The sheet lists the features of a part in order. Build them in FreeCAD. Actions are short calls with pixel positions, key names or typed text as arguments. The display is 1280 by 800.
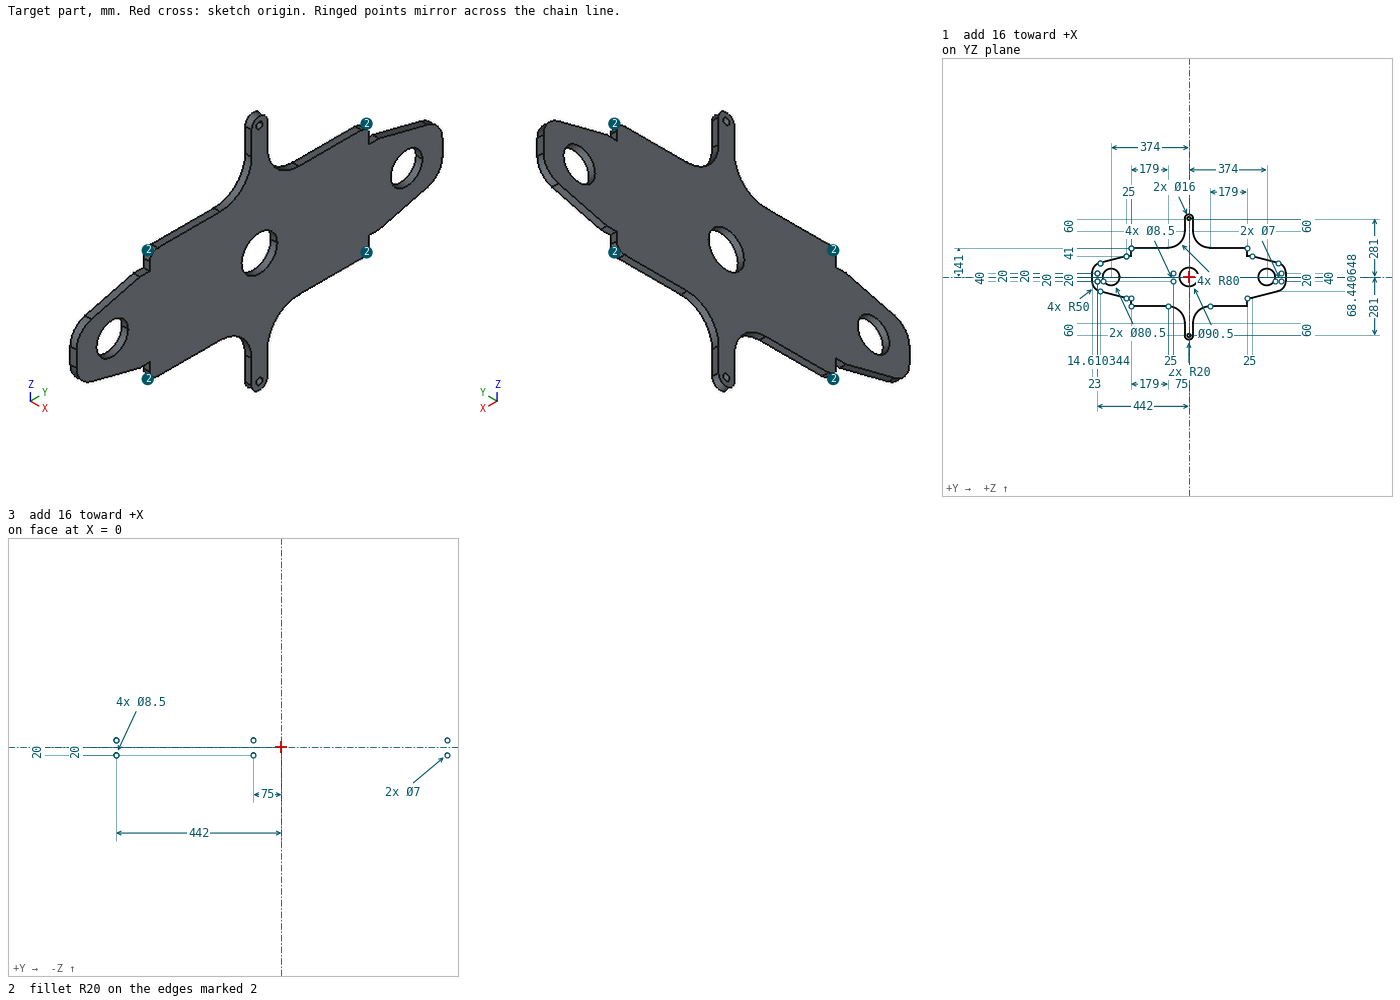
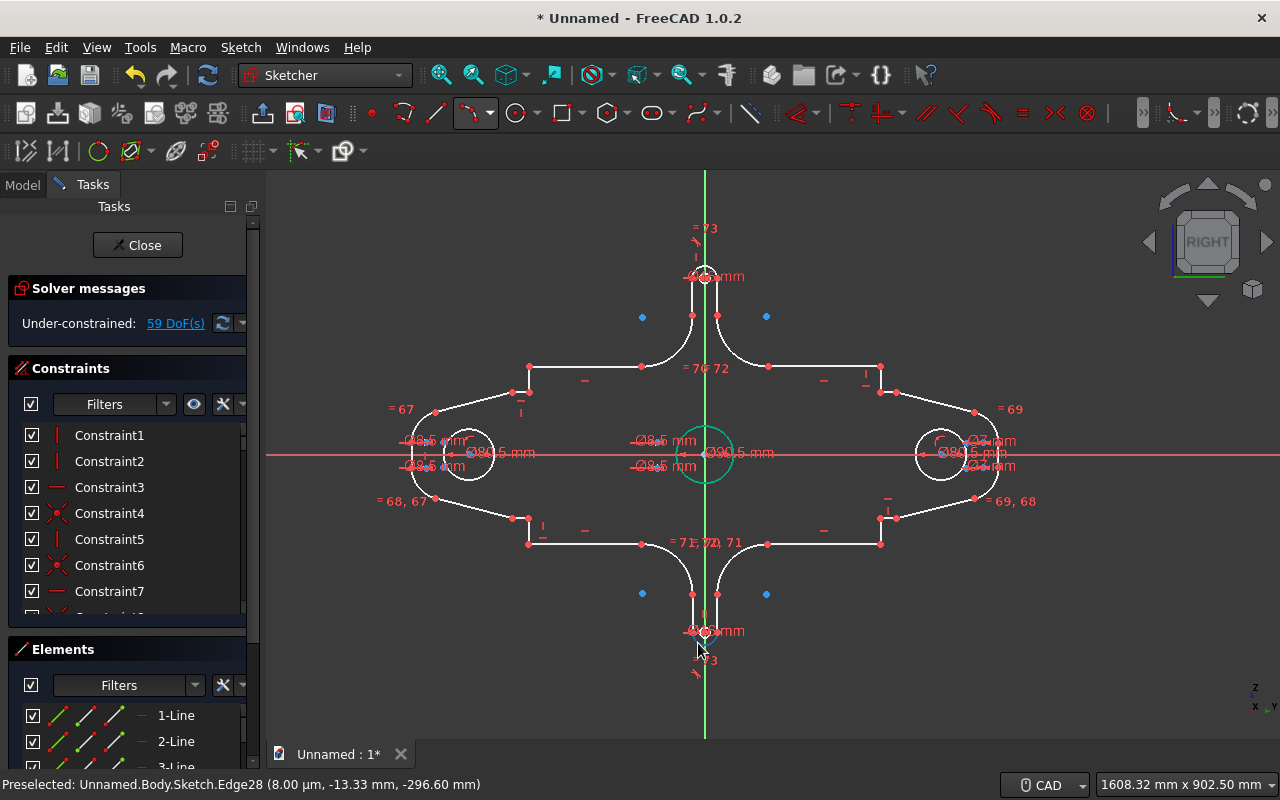
click(705, 278)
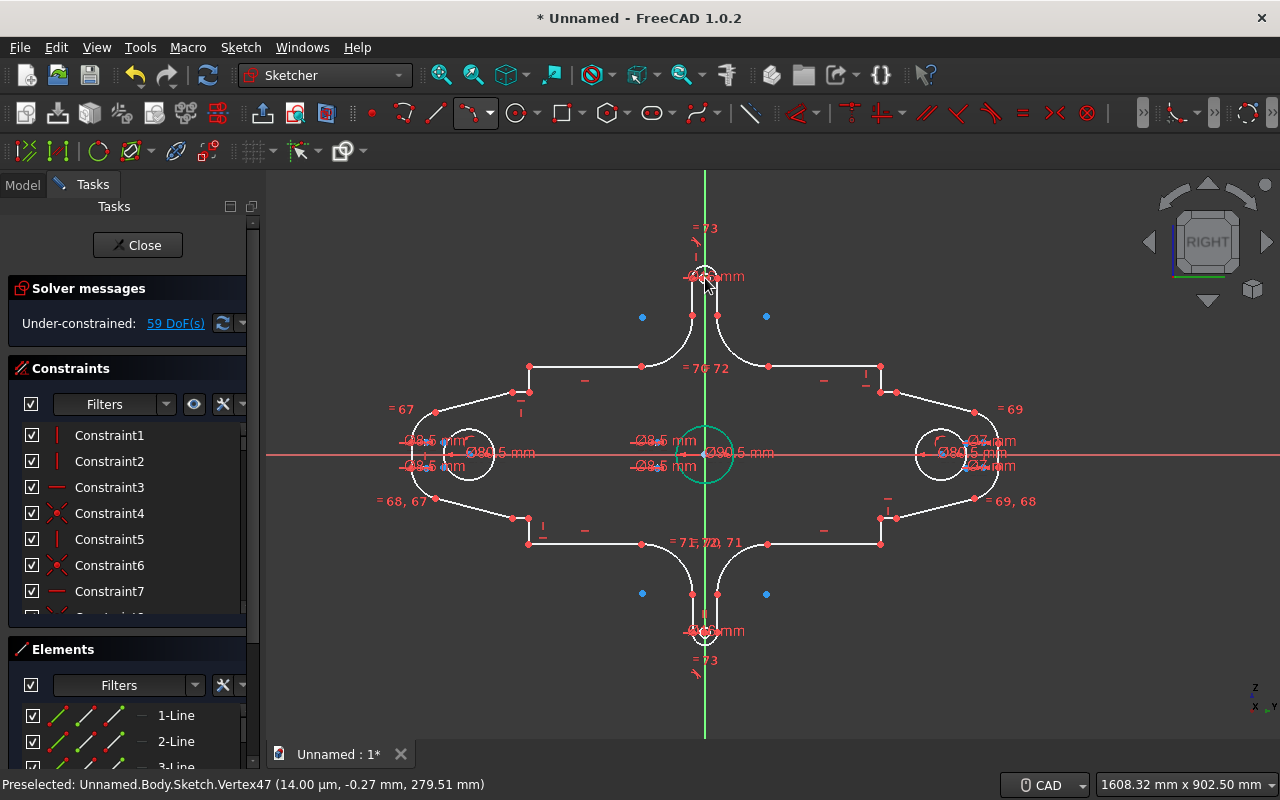
click(705, 528)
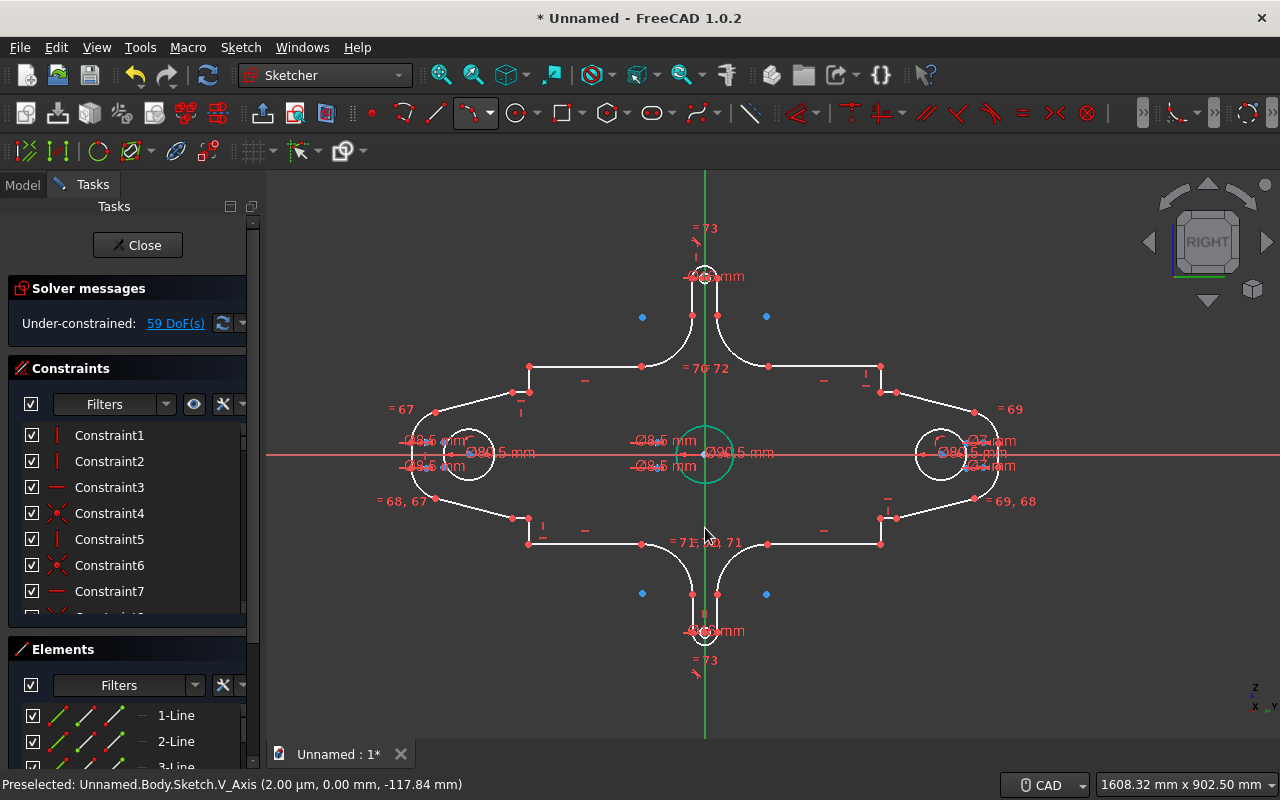
click(850, 114)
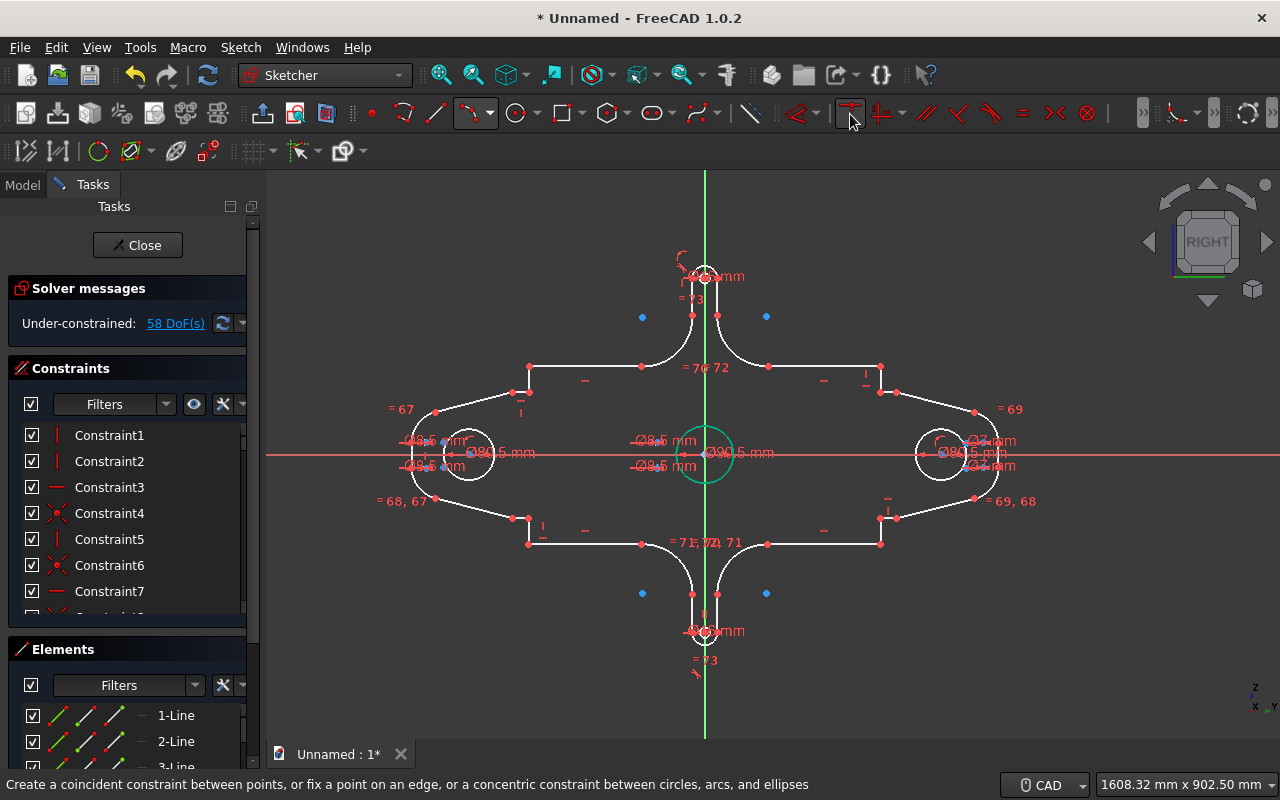
click(705, 633)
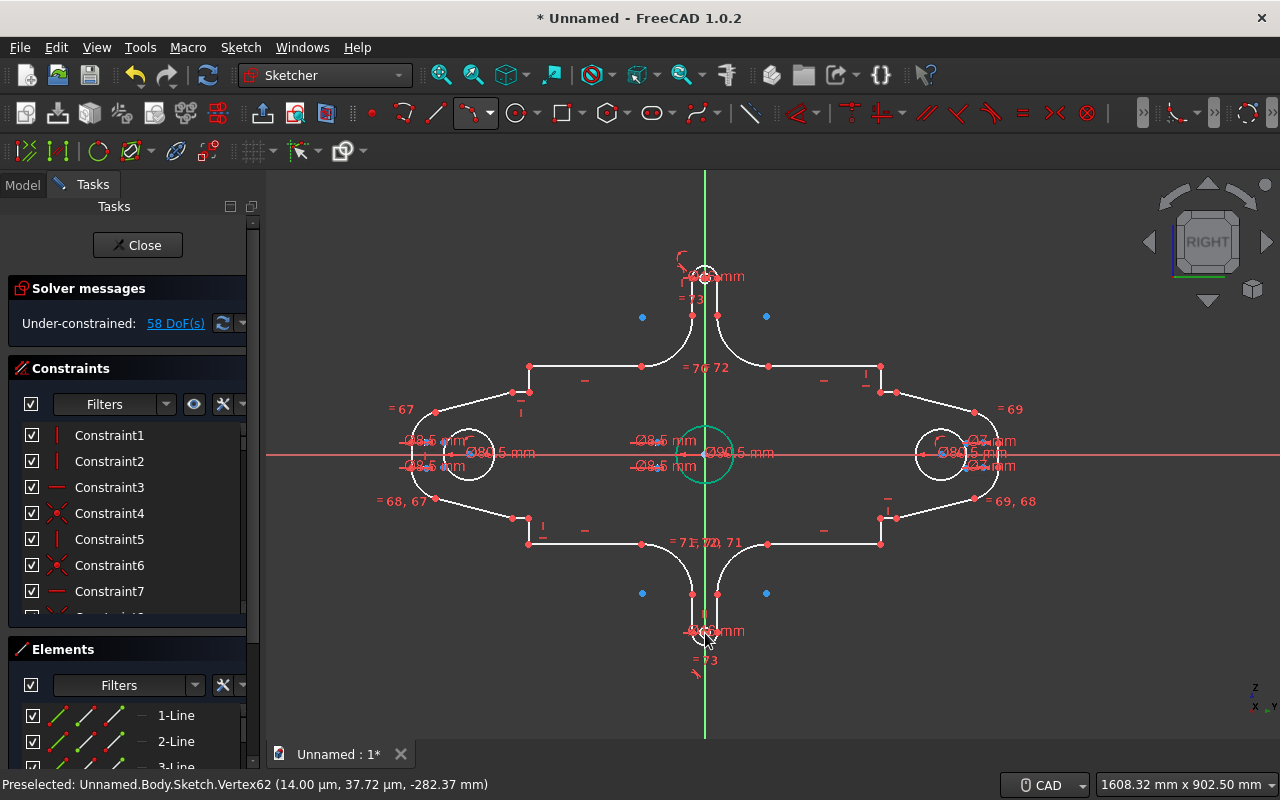
click(705, 528)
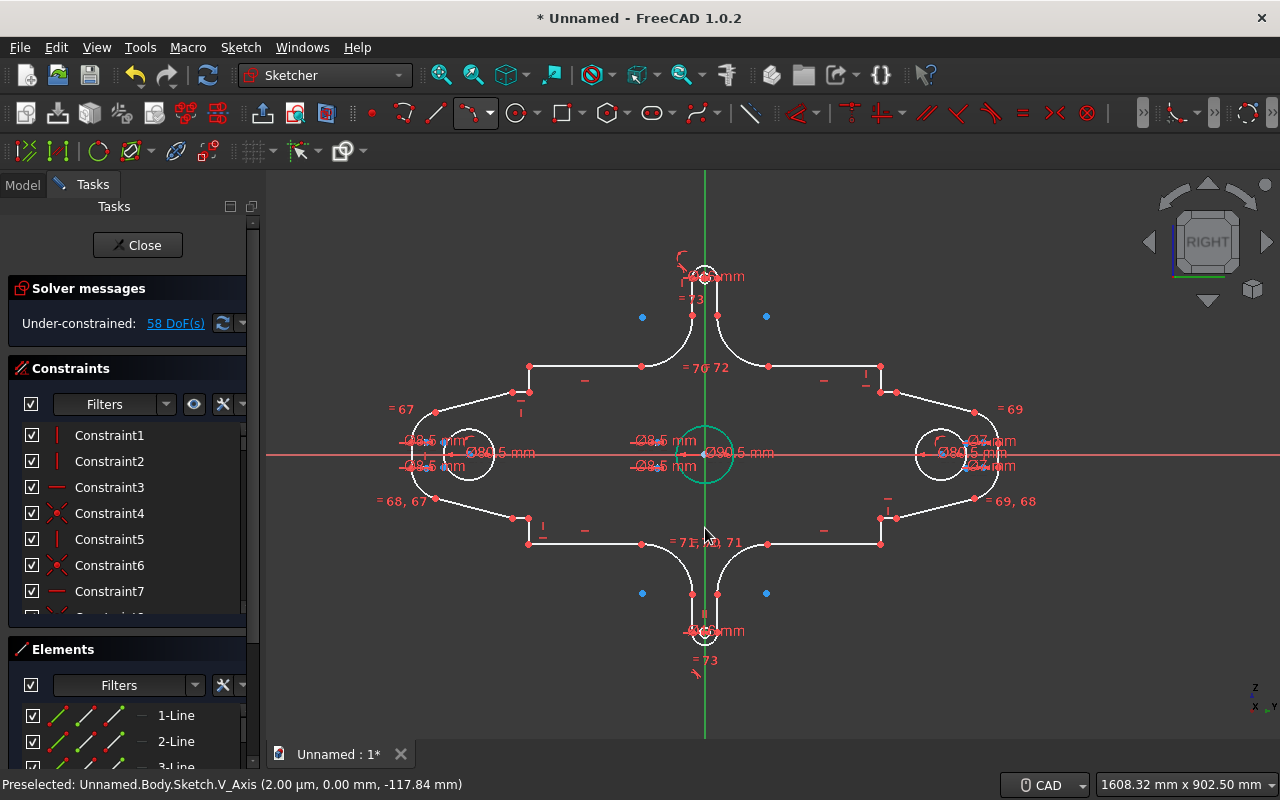
click(850, 114)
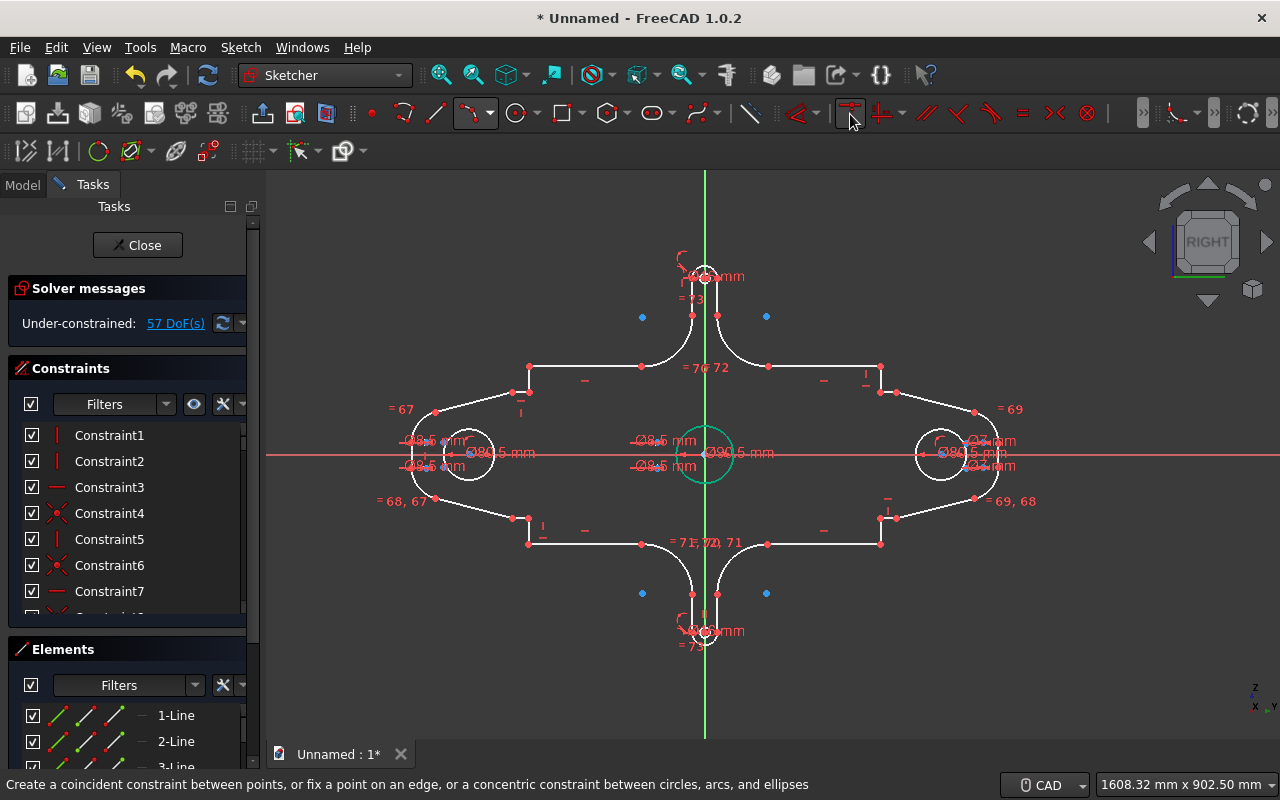
click(443, 468)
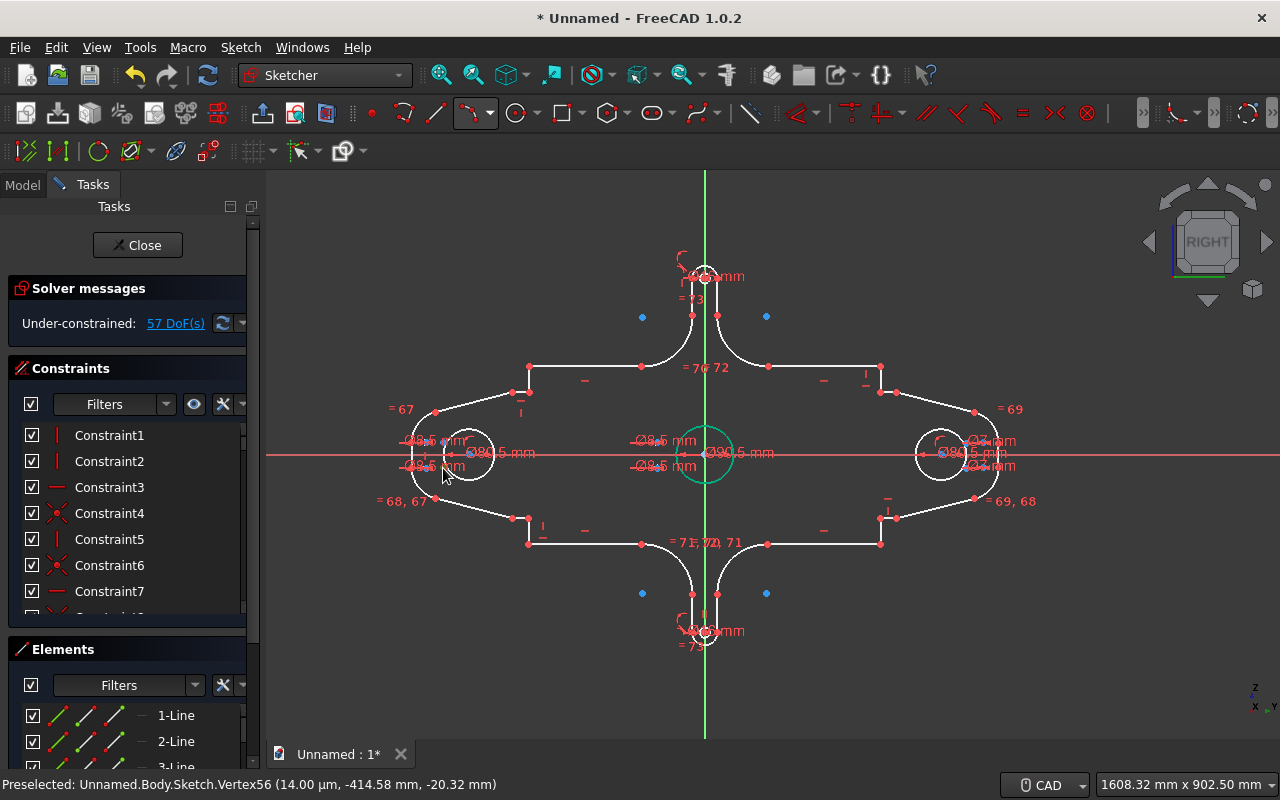
click(967, 468)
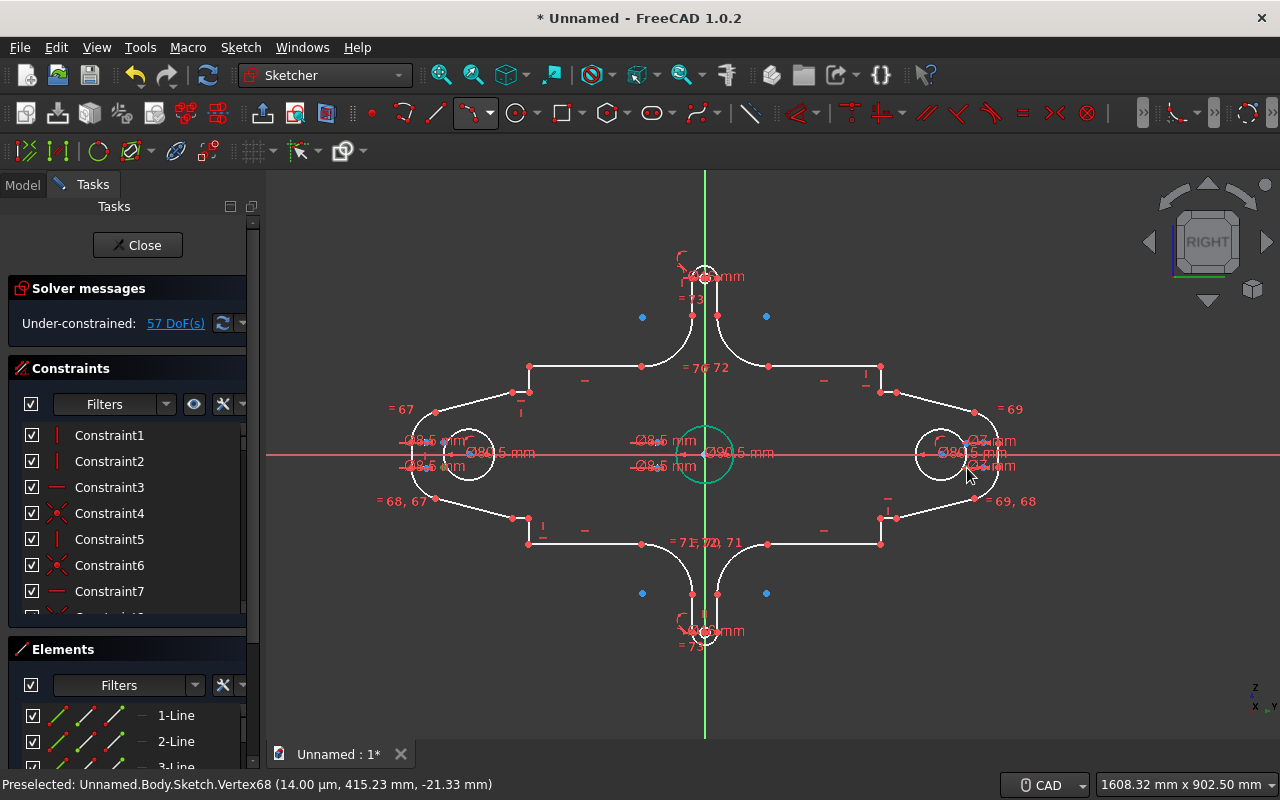
click(705, 528)